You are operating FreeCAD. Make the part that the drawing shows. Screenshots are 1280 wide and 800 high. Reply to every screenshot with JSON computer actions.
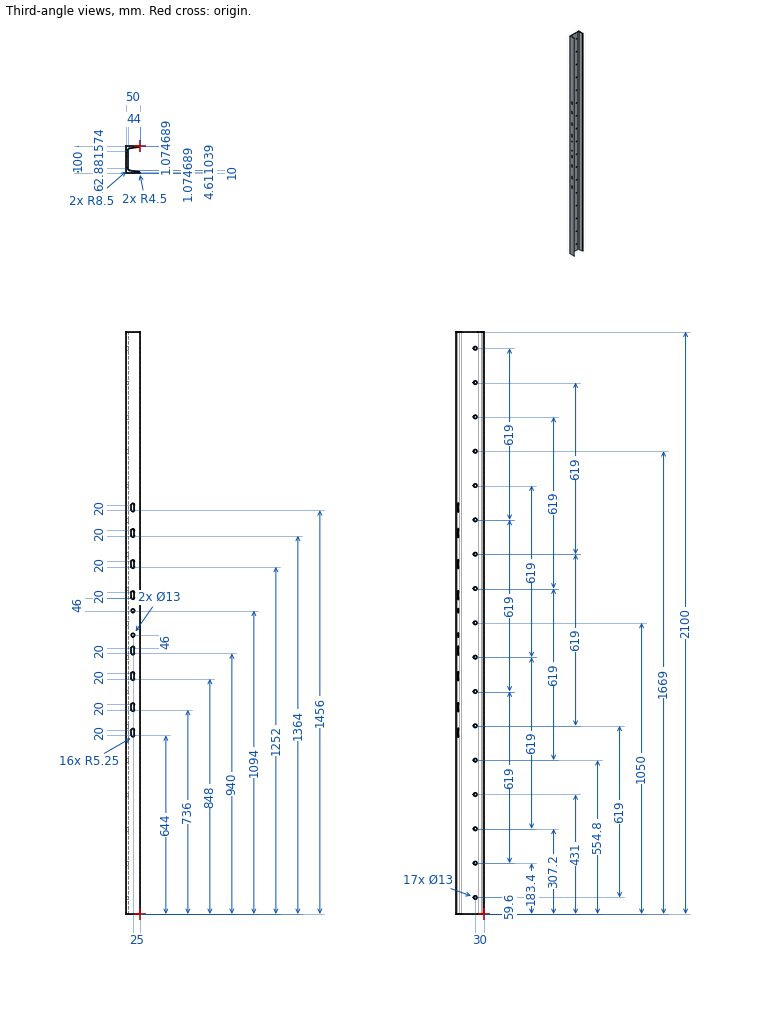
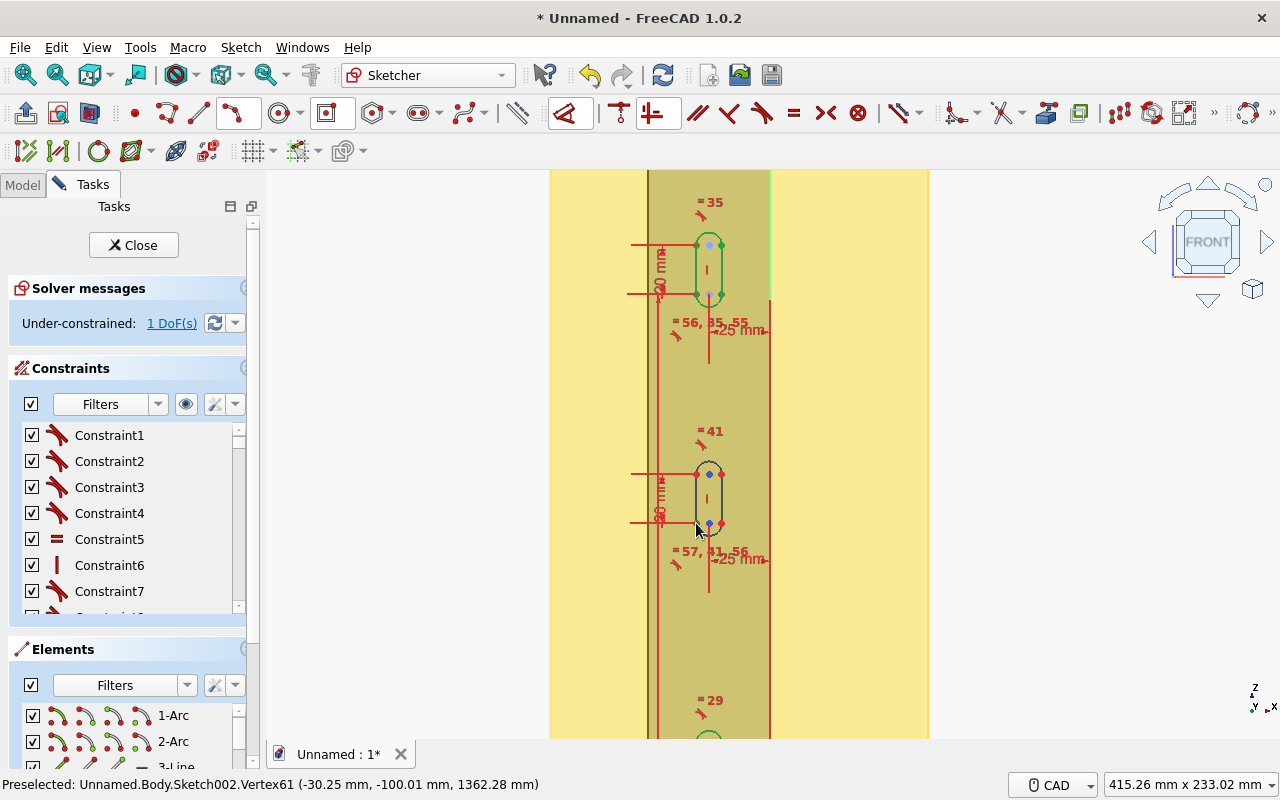
{"action": "key", "text": "i"}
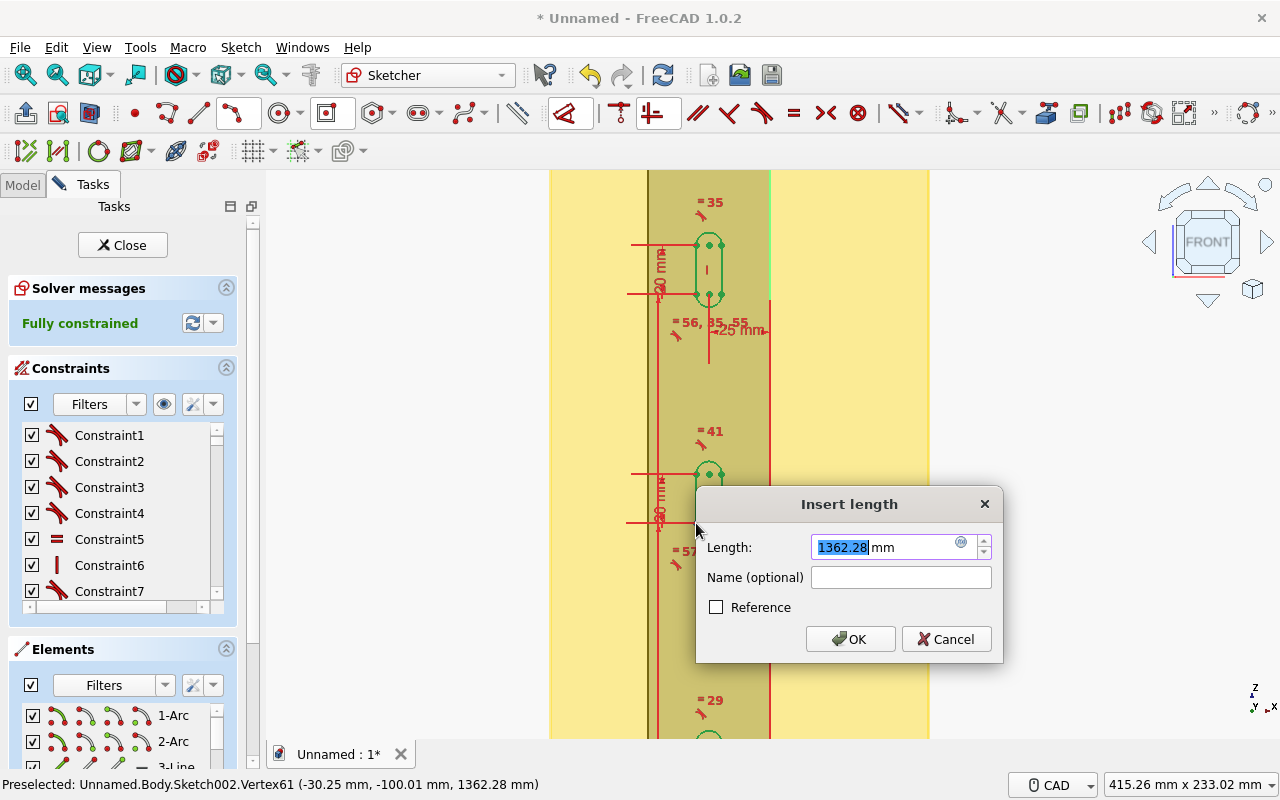
{"action": "type", "text": "1364"}
{"action": "key", "text": "Return"}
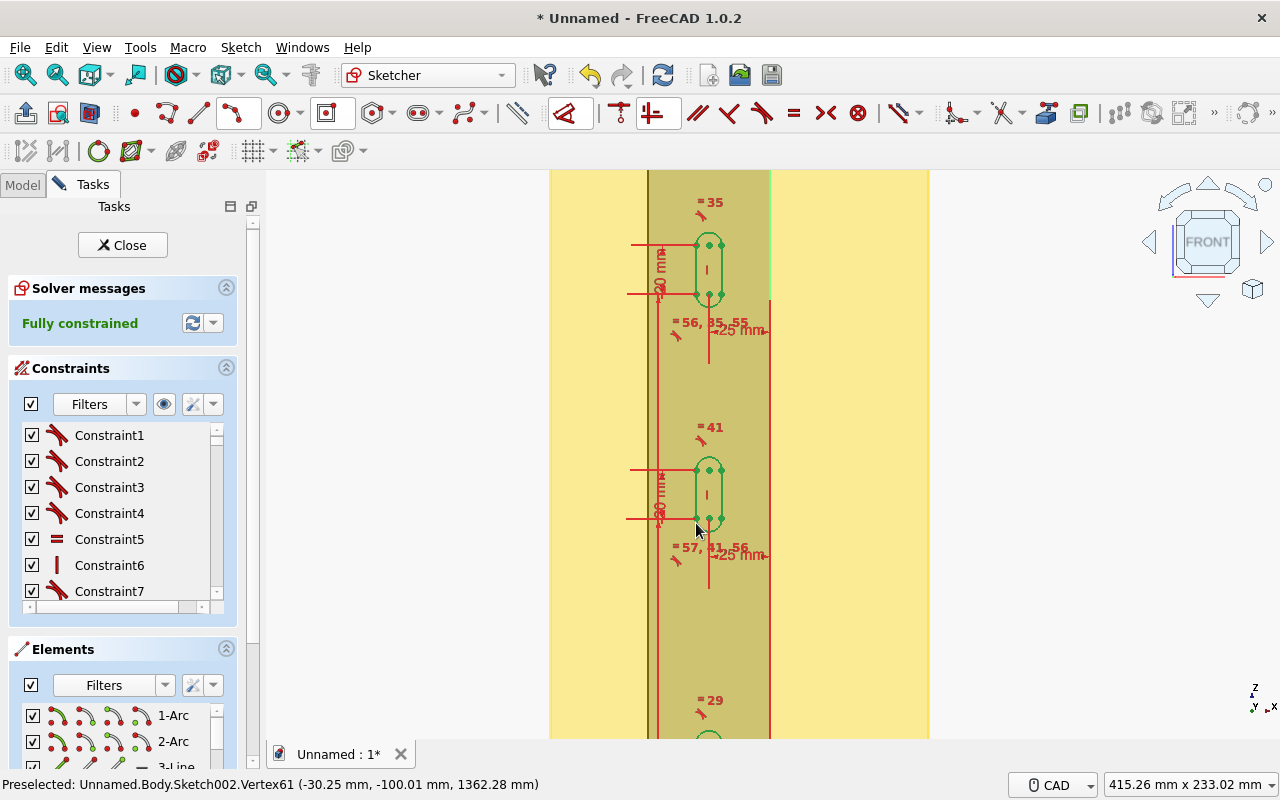
{"action": "left_click", "coordinate": [123, 245]}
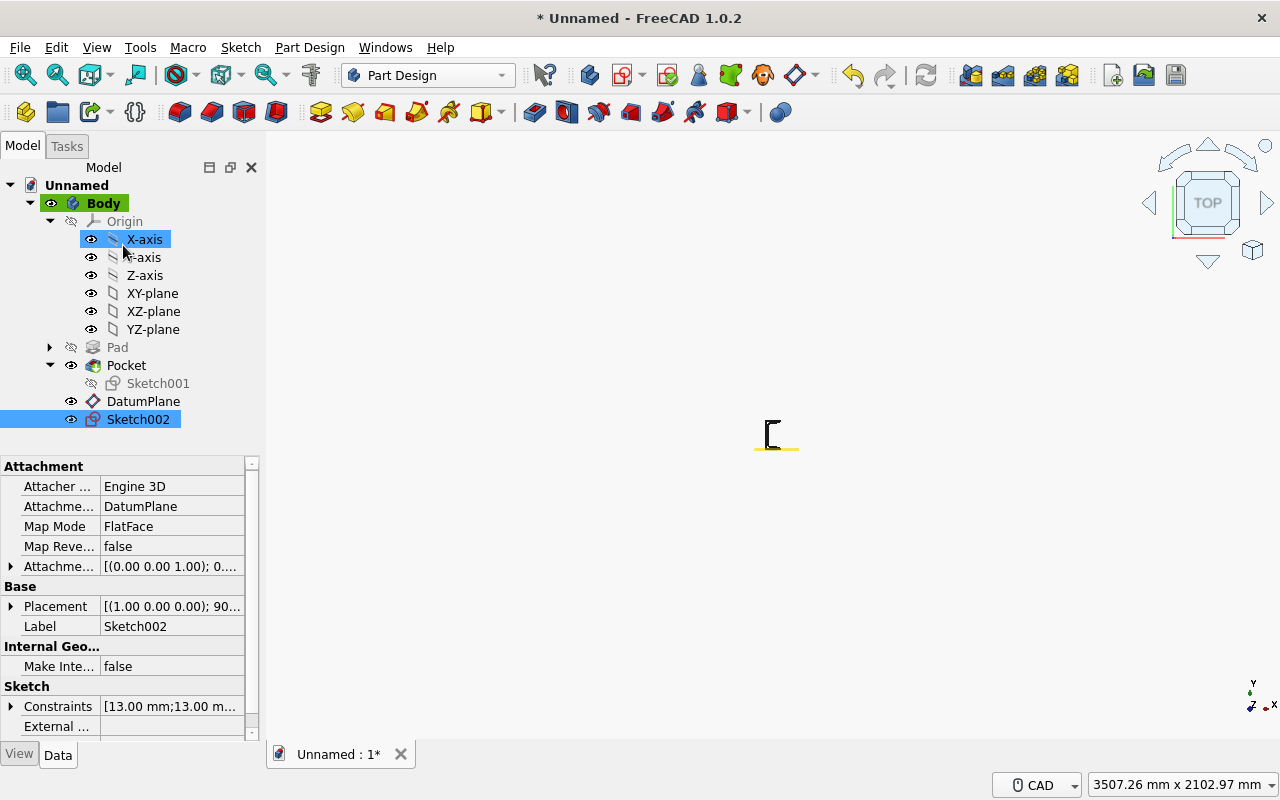
{"action": "left_click", "coordinate": [536, 112]}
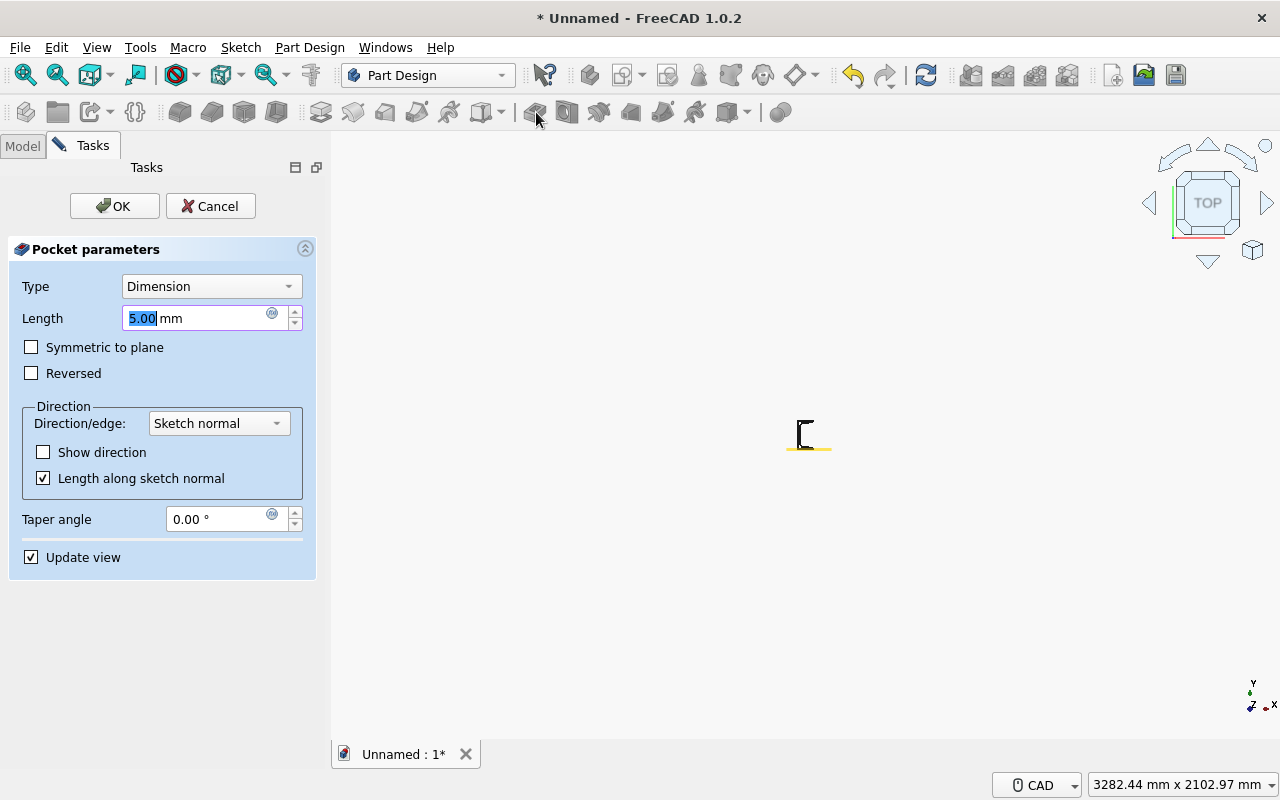
{"action": "type", "text": "10"}
{"action": "key", "text": "Tab"}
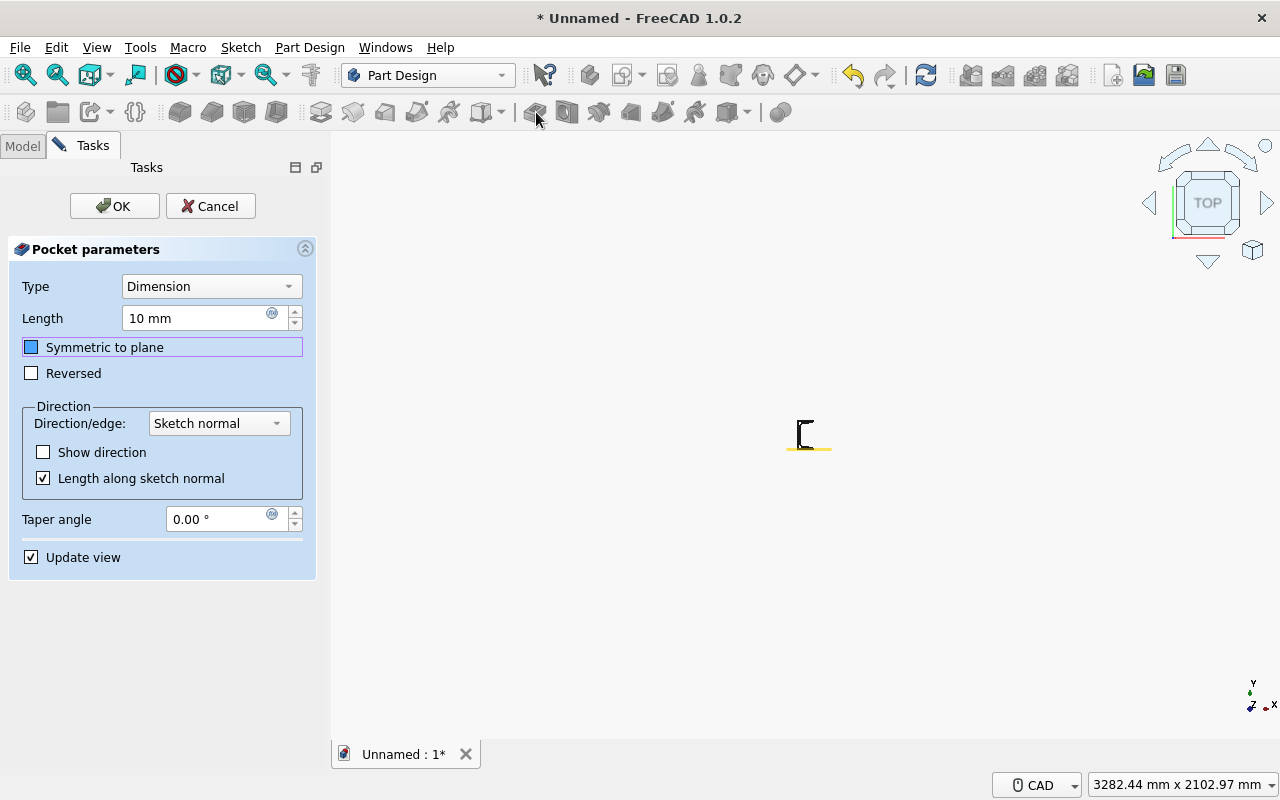
{"action": "left_click", "coordinate": [115, 206]}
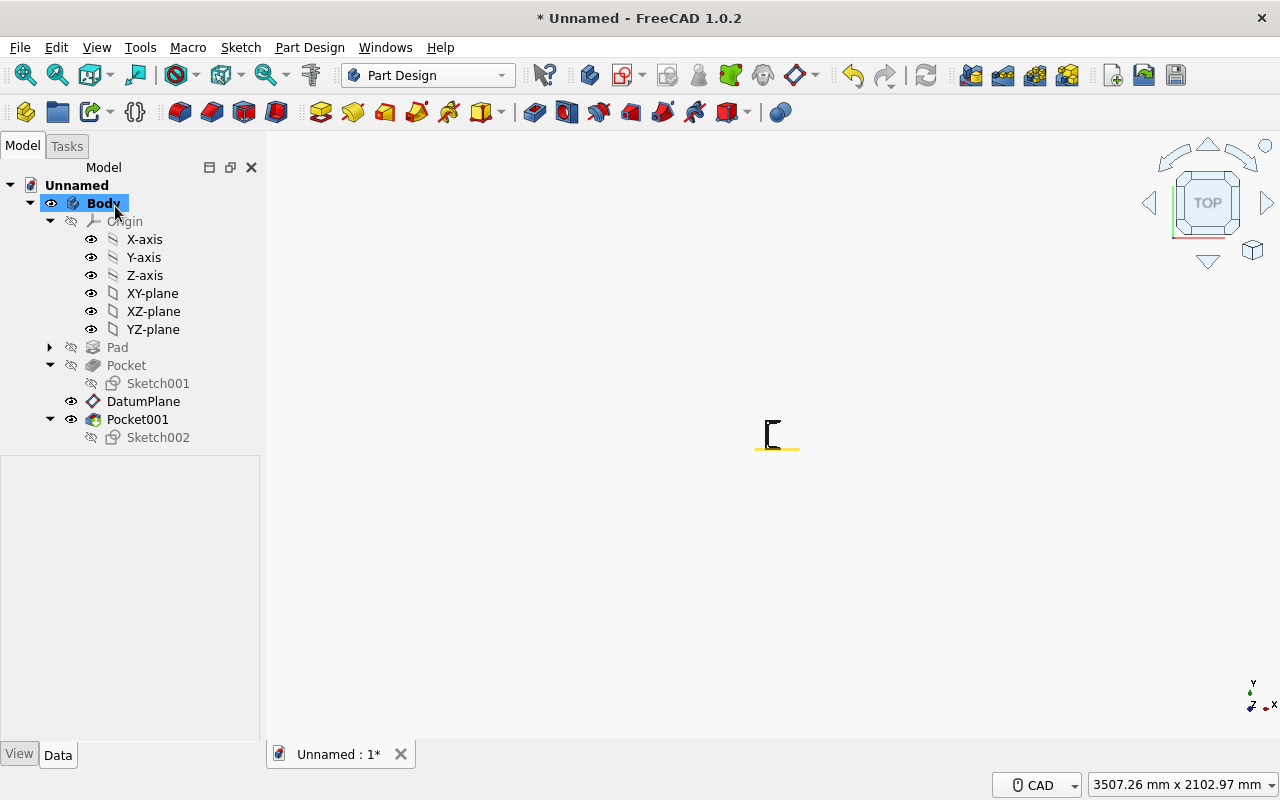
{"action": "left_click", "coordinate": [116, 401]}
{"action": "key", "text": "space"}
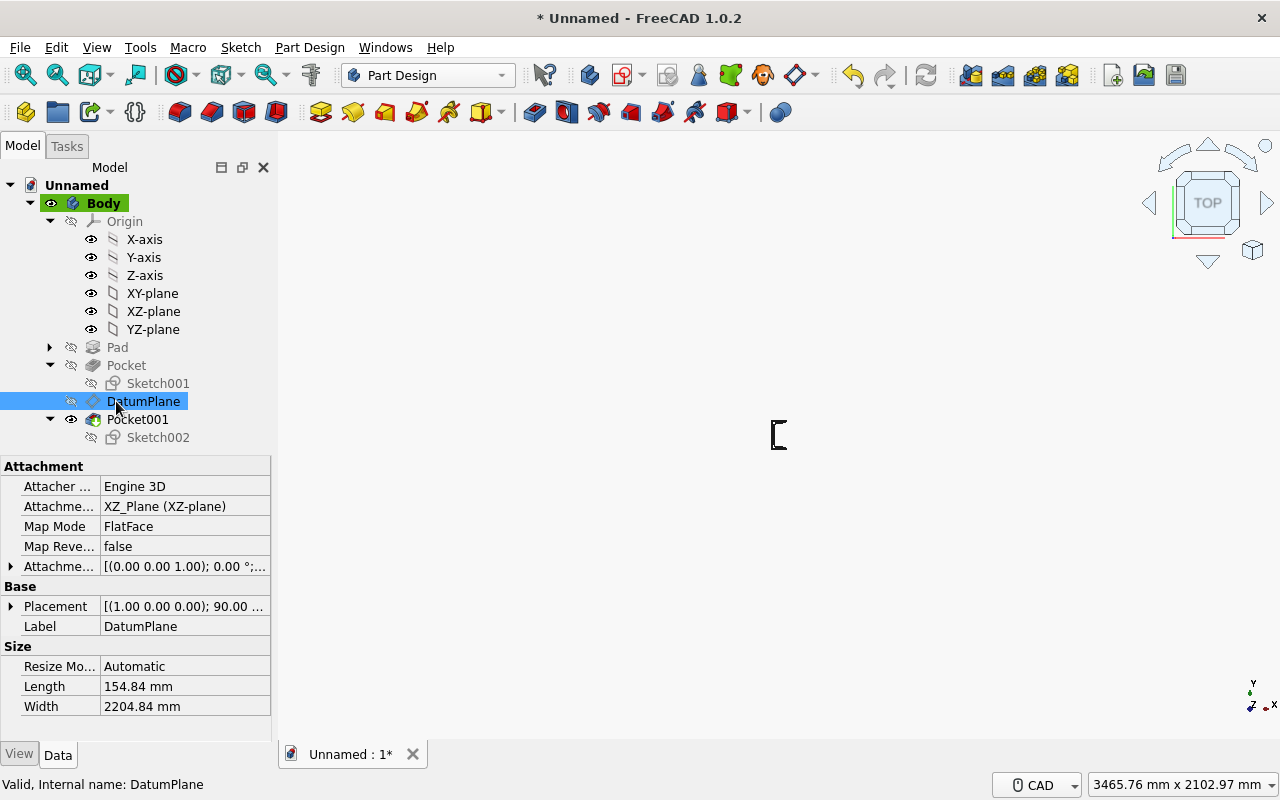
{"action": "key", "text": "0"}